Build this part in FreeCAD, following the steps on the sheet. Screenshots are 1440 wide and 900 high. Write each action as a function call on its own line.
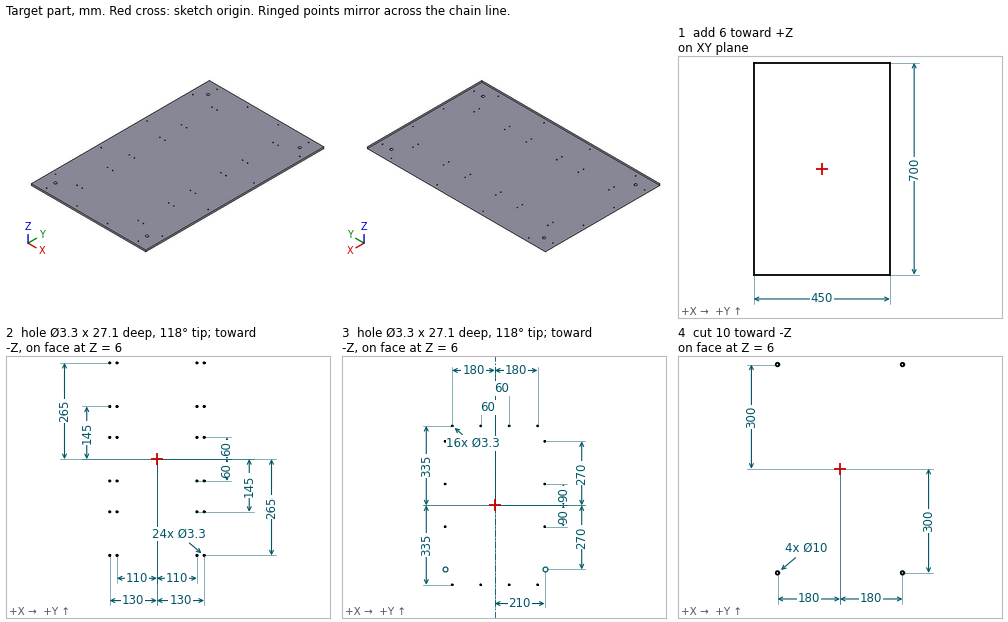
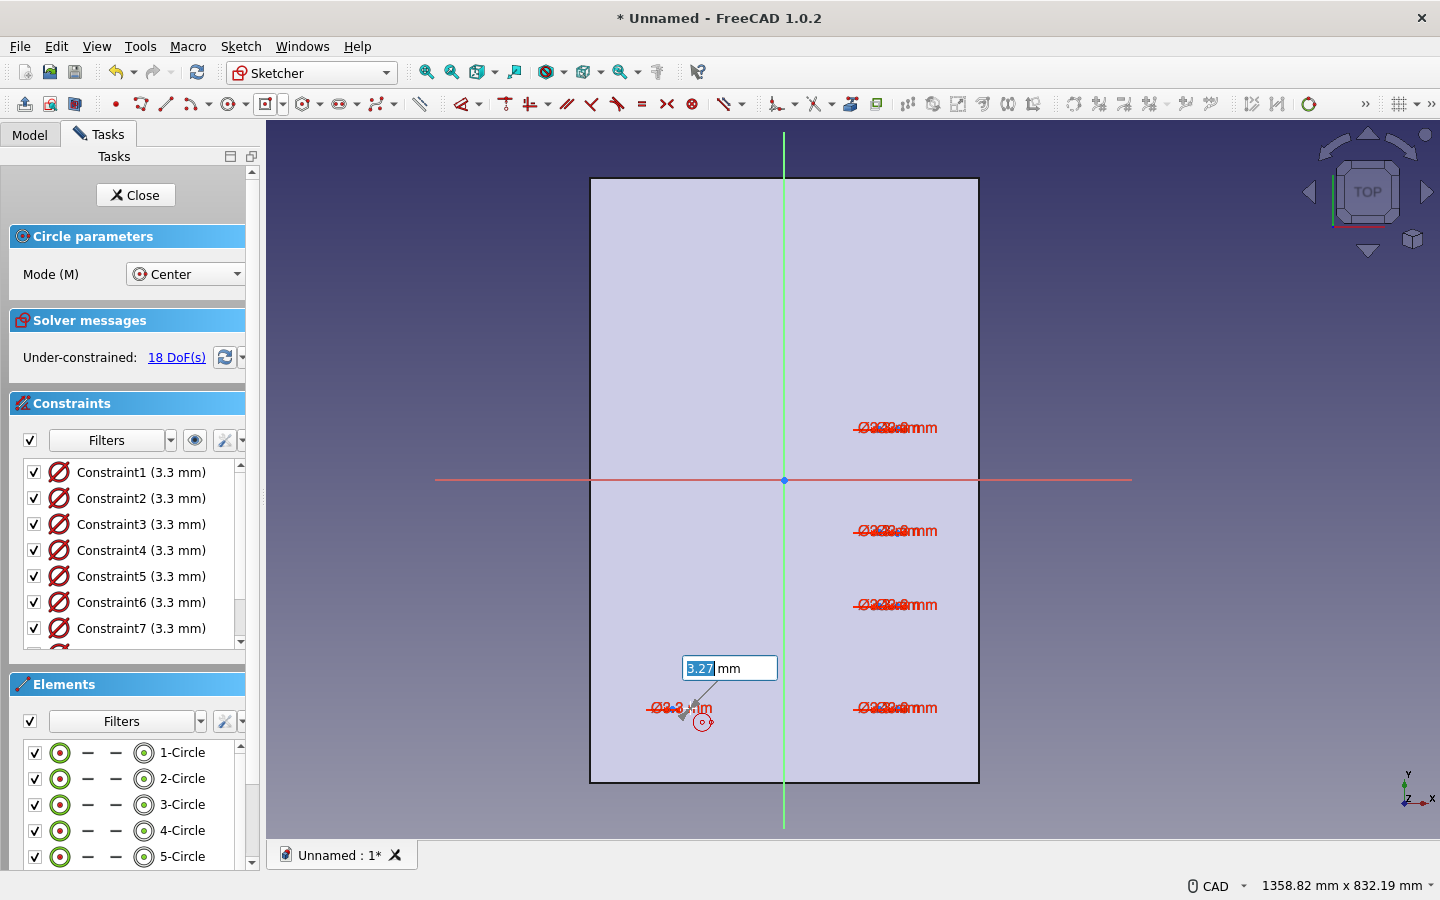
text(3.3)
key(Return)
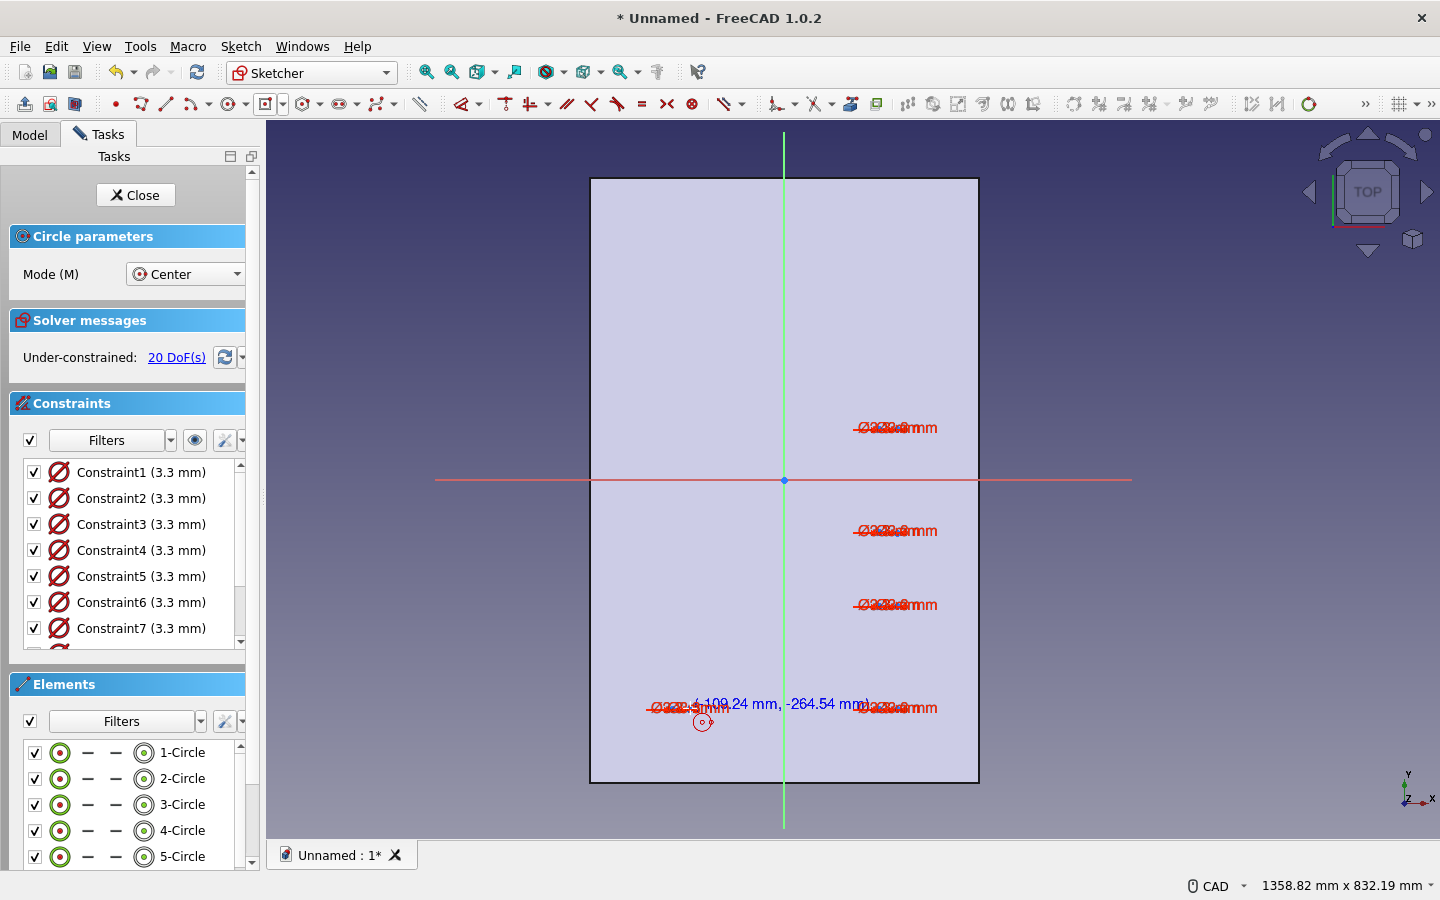
scroll(672, 606, up, 14)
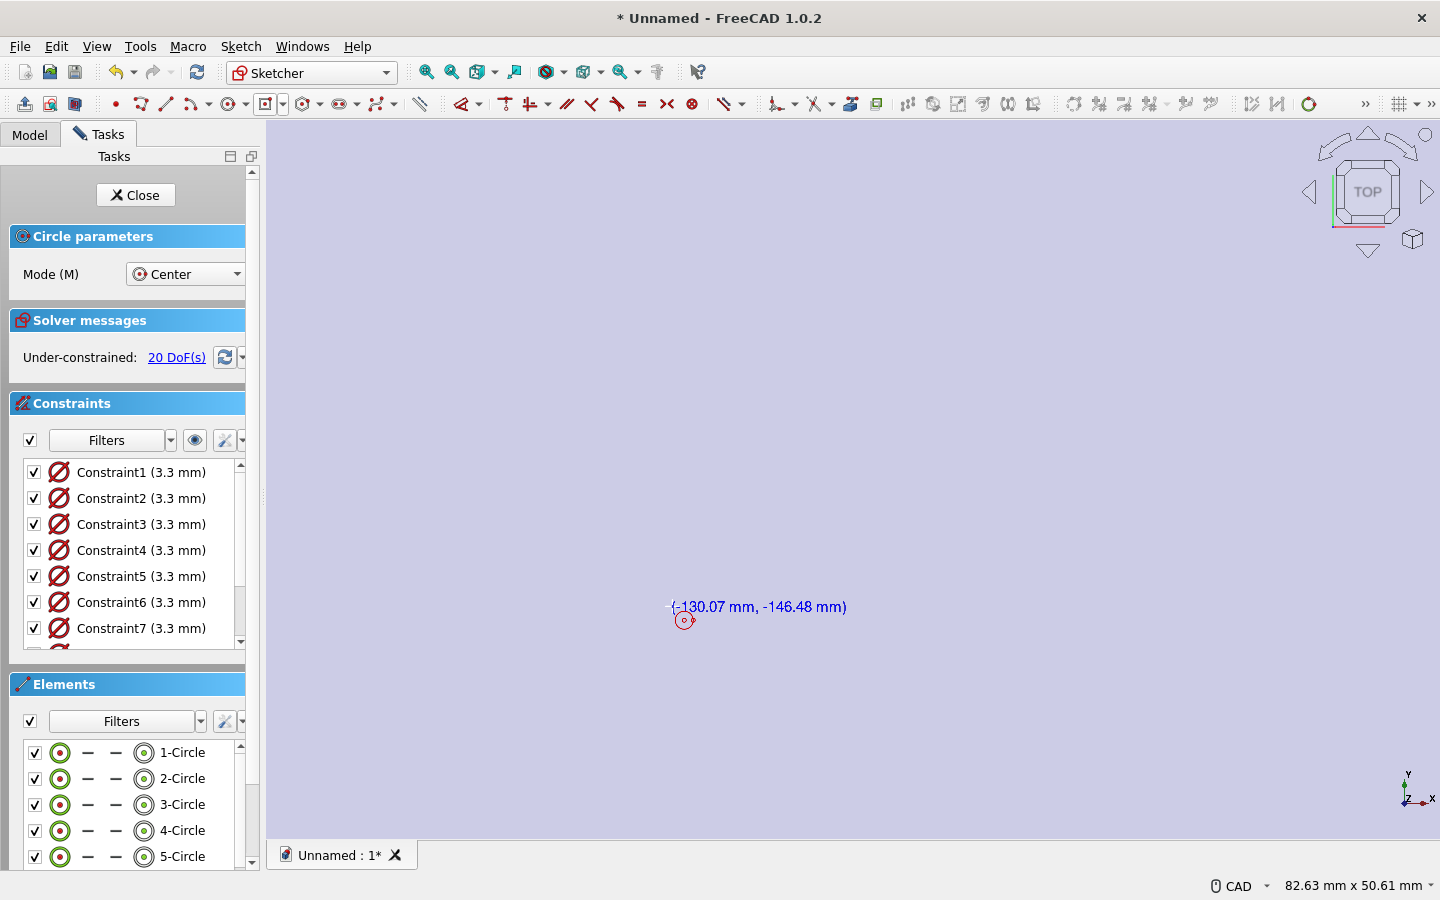
scroll(672, 606, down, 14)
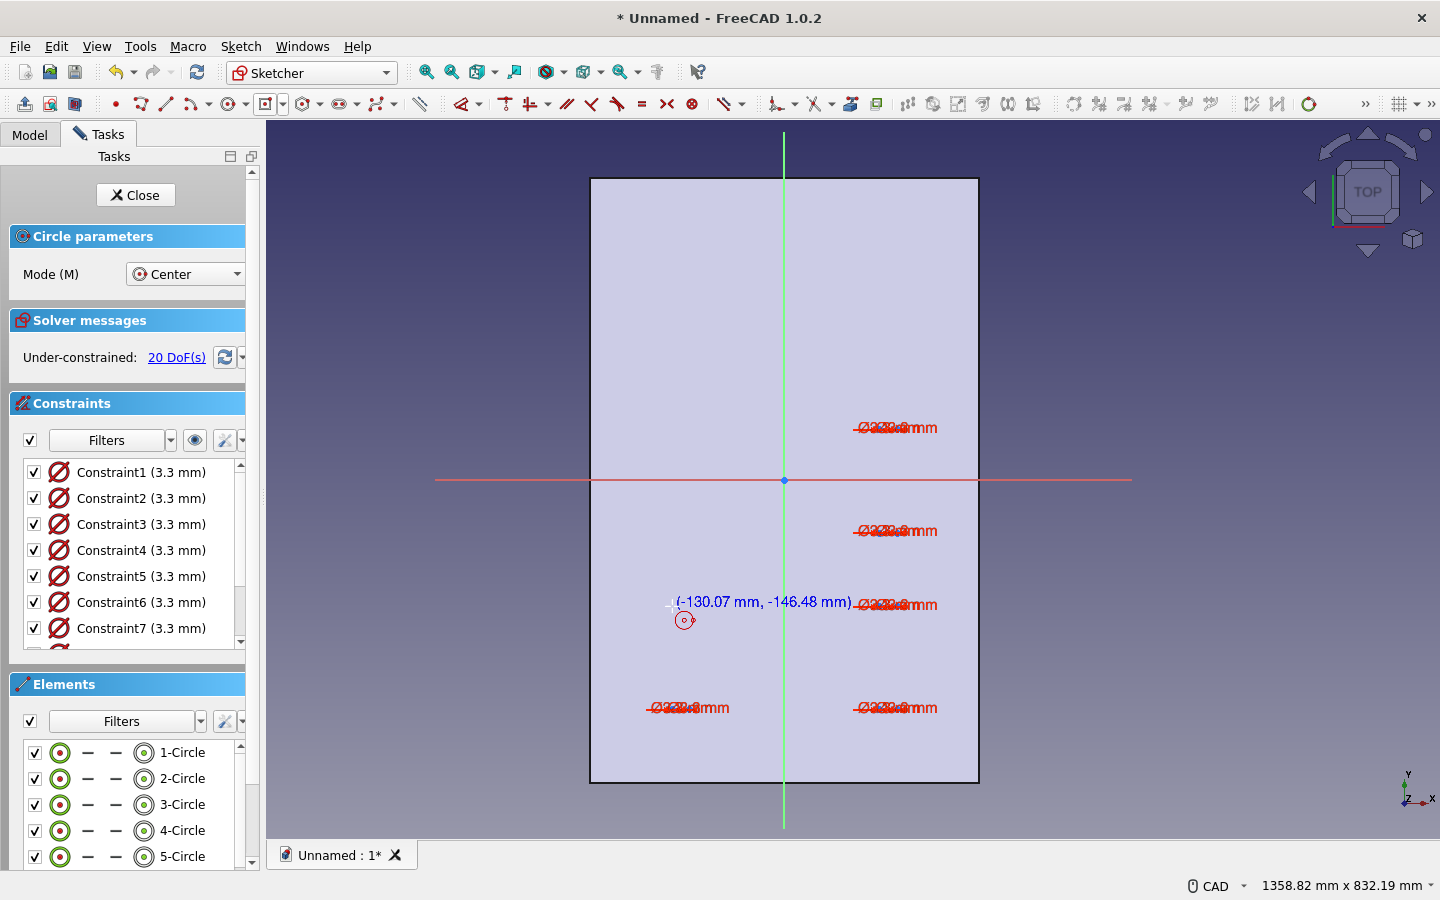
click(672, 606)
move(673, 605)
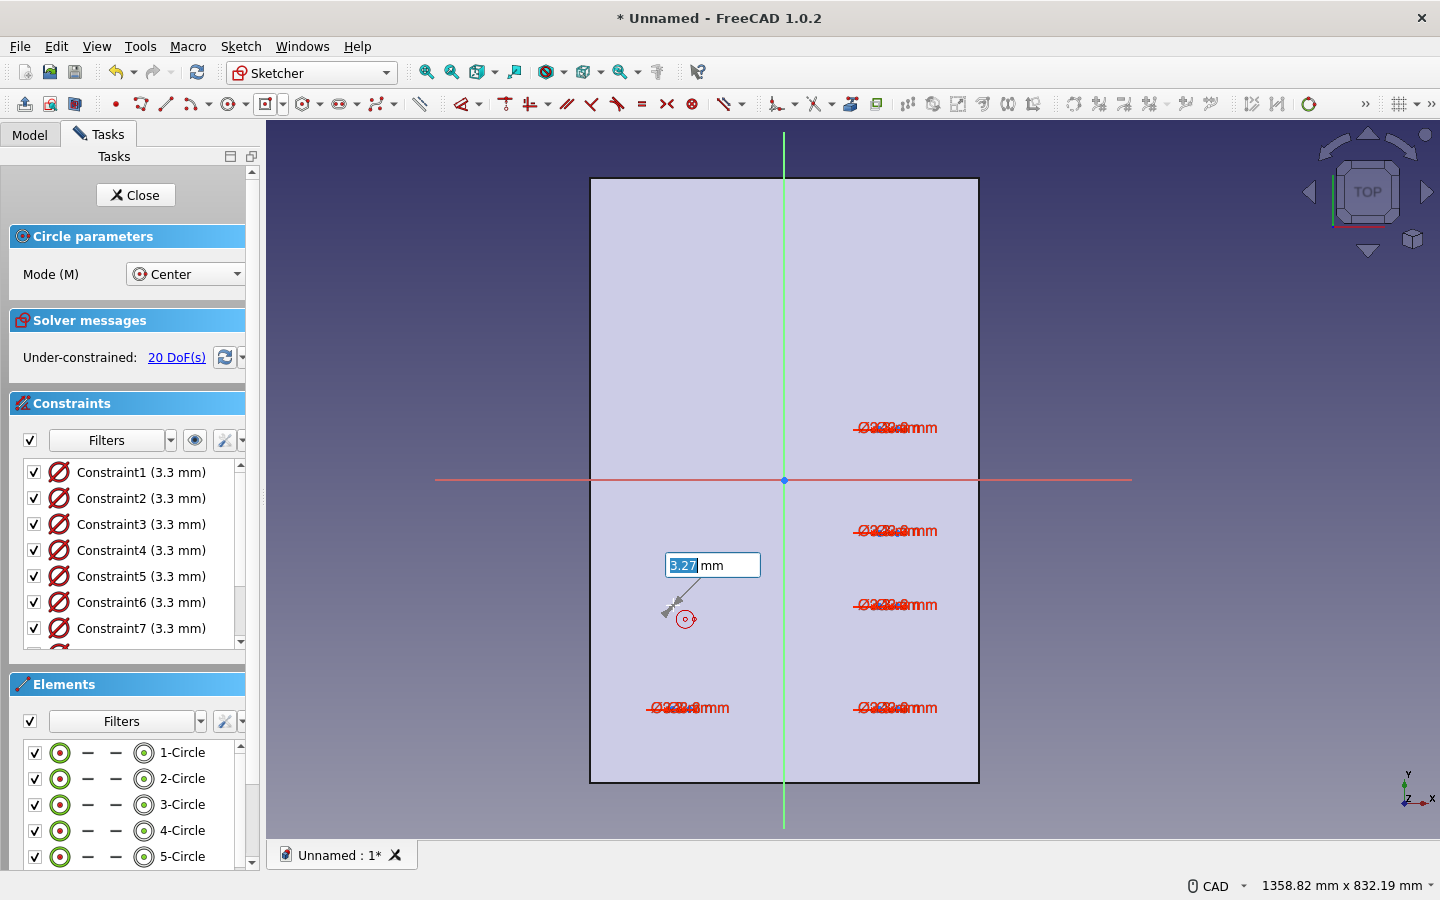
text(3.3)
key(Return)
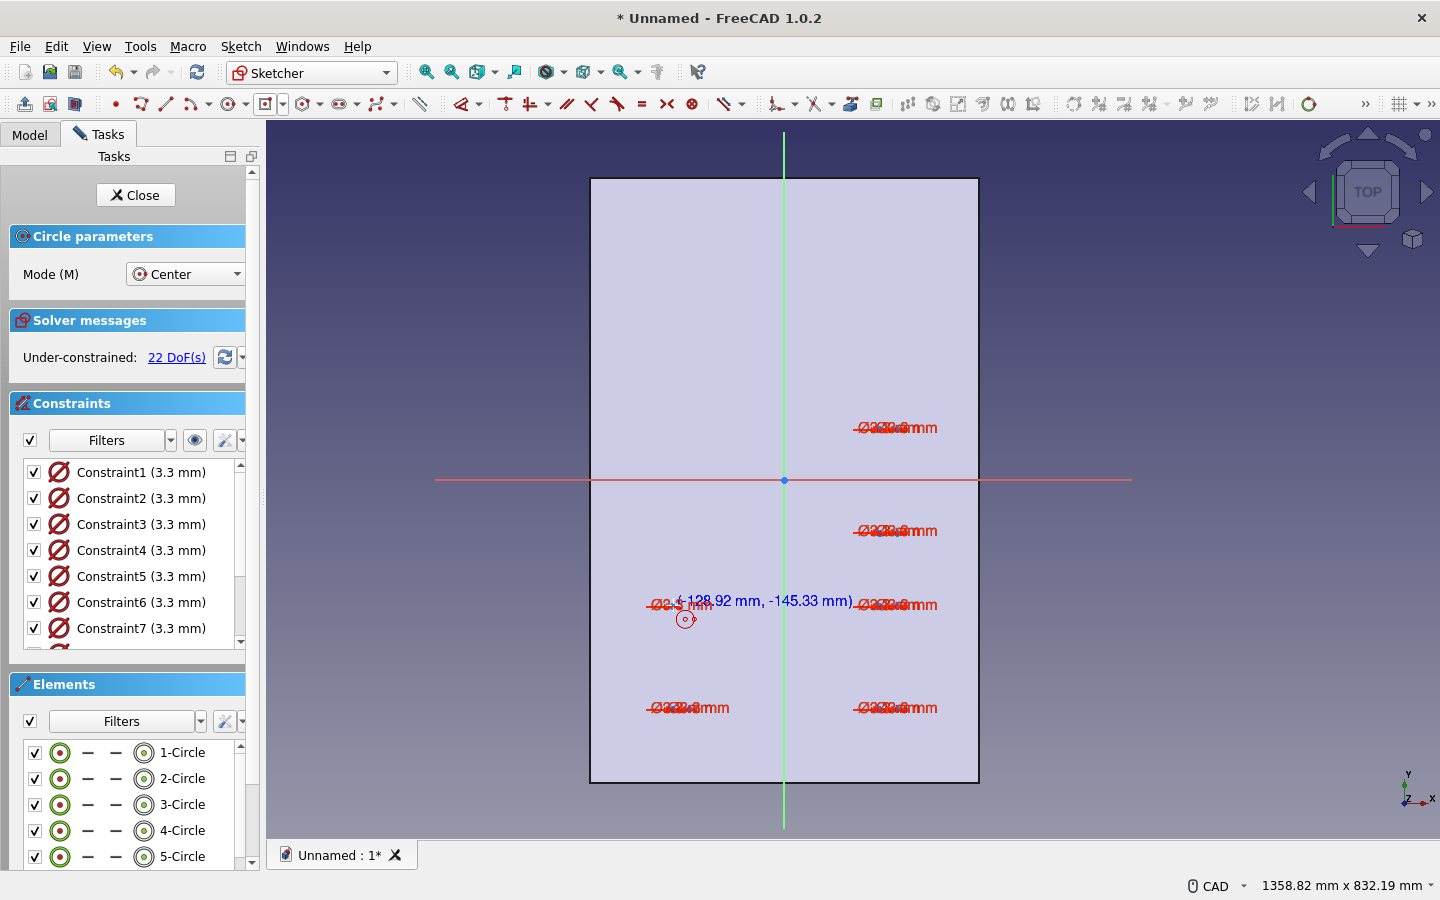
scroll(689, 606, up, 14)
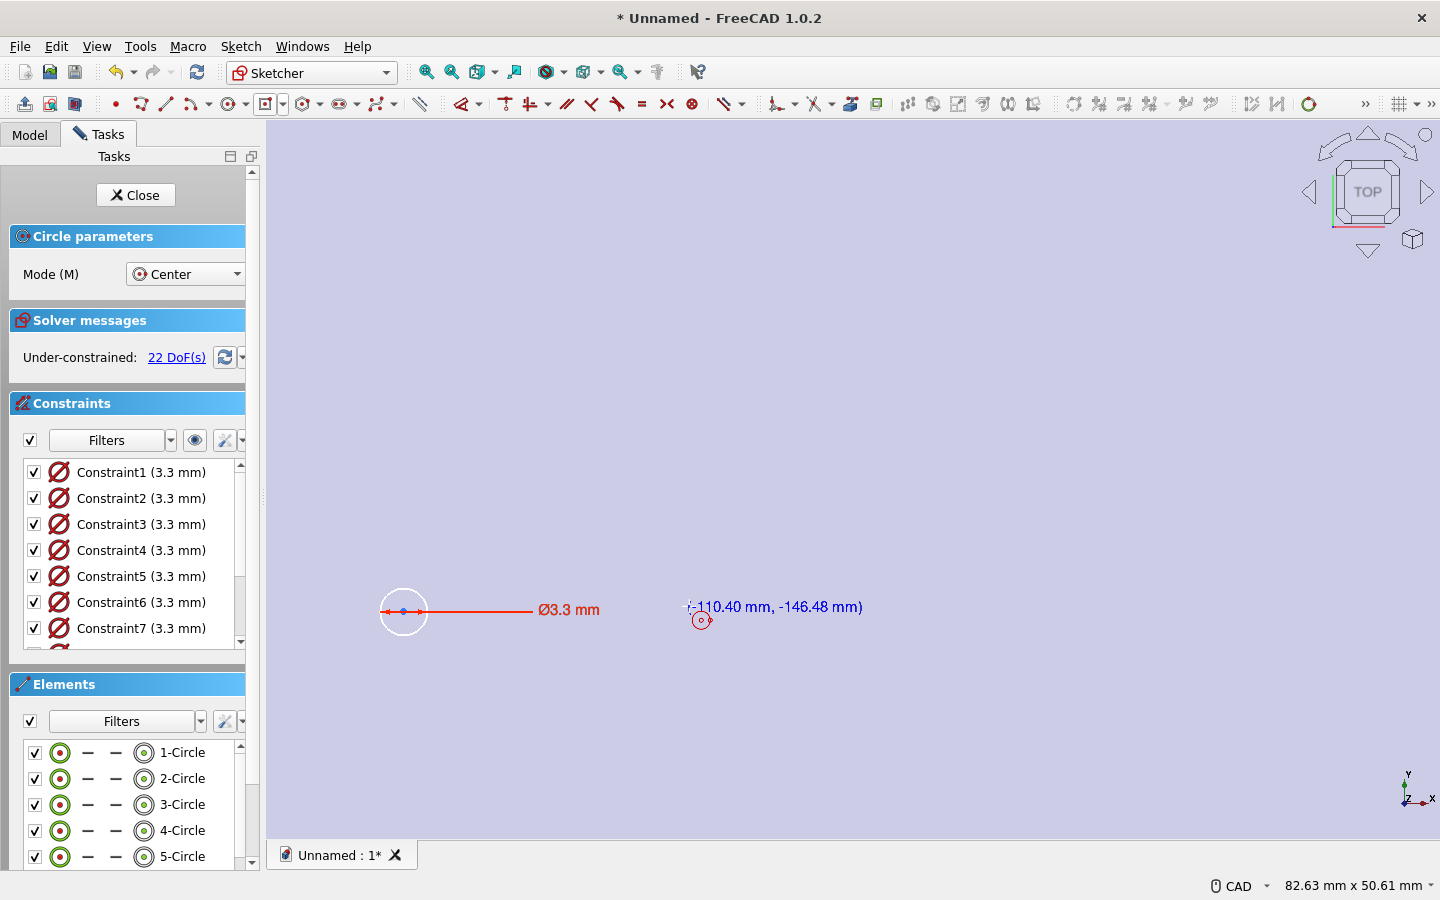
scroll(689, 606, down, 14)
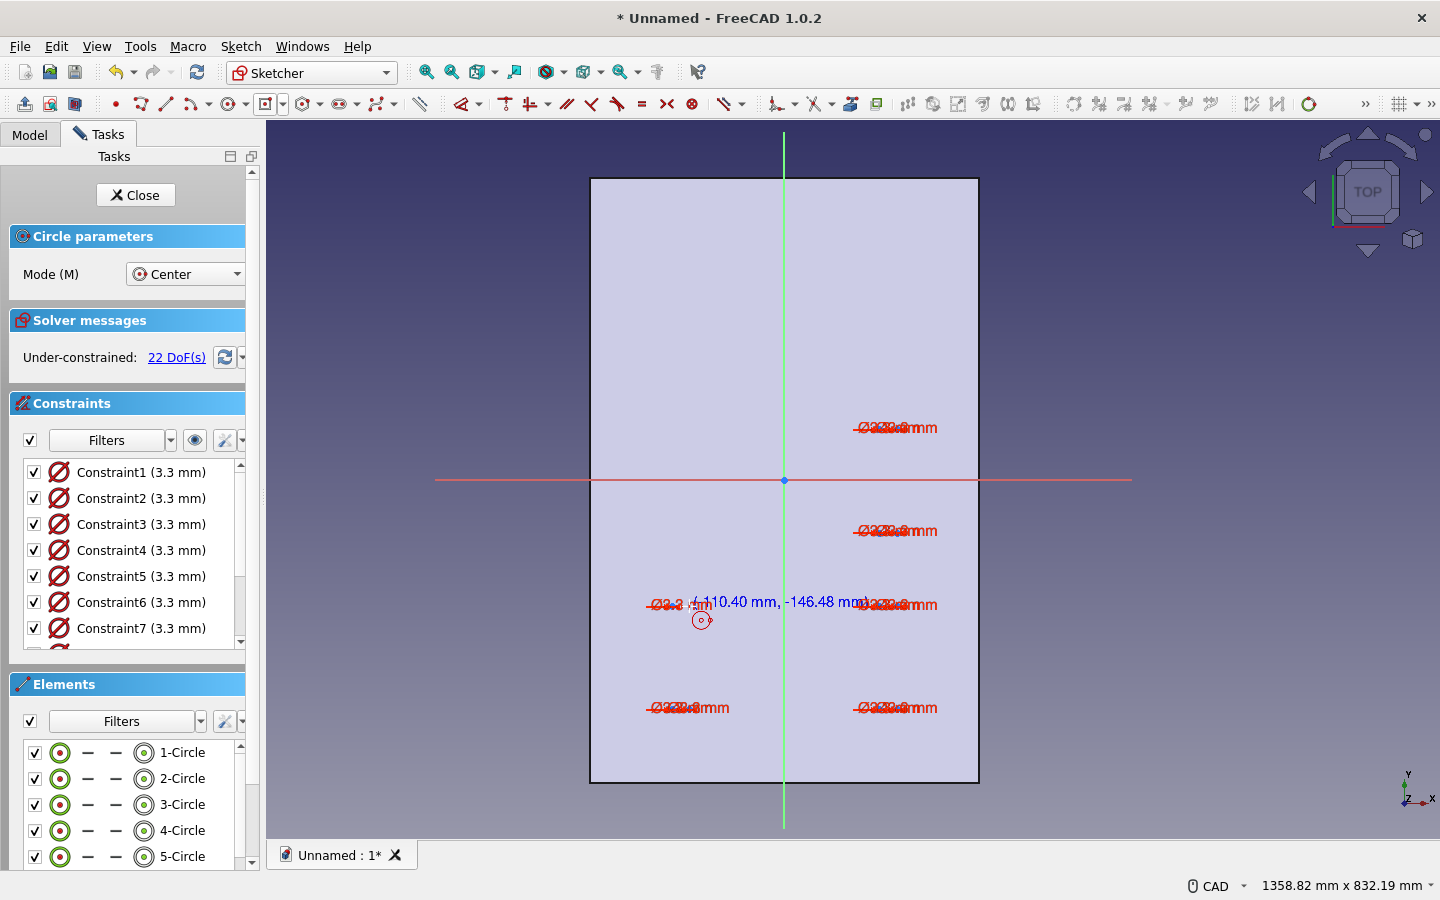
click(689, 606)
move(690, 605)